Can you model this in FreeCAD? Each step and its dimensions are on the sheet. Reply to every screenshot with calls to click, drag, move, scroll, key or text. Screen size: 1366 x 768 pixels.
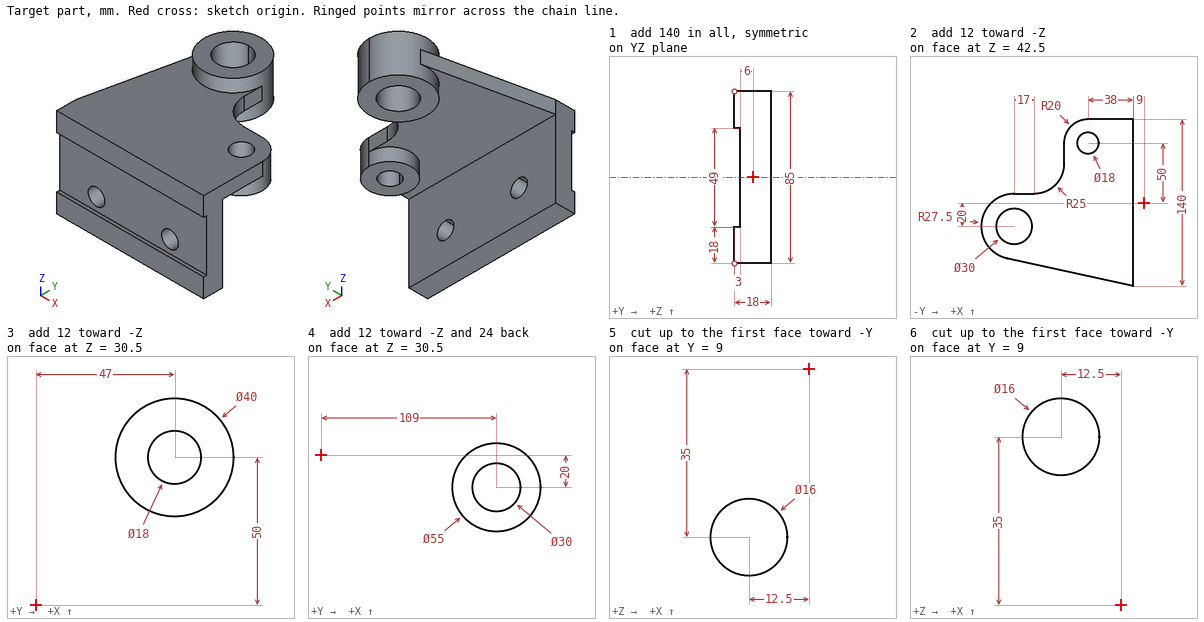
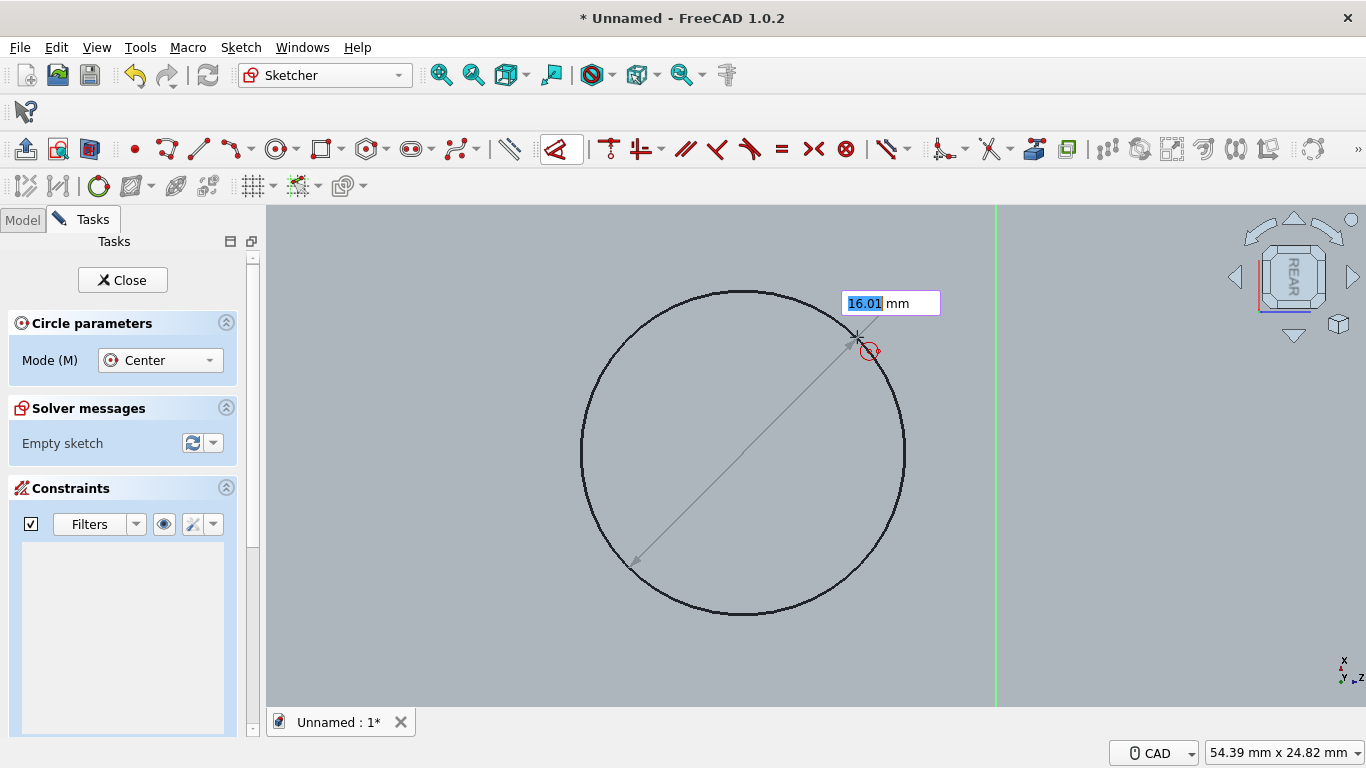
text(16)
key(Return)
key(Escape)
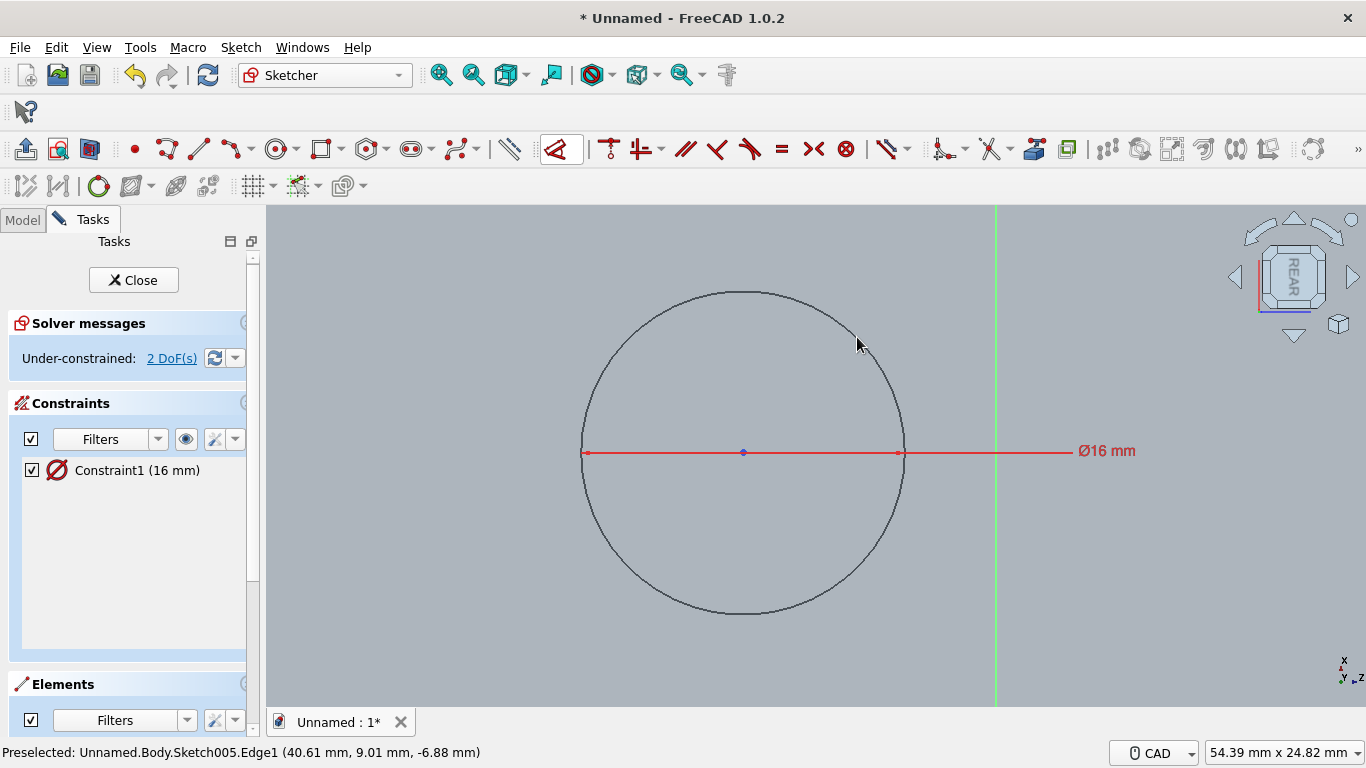
click(743, 453)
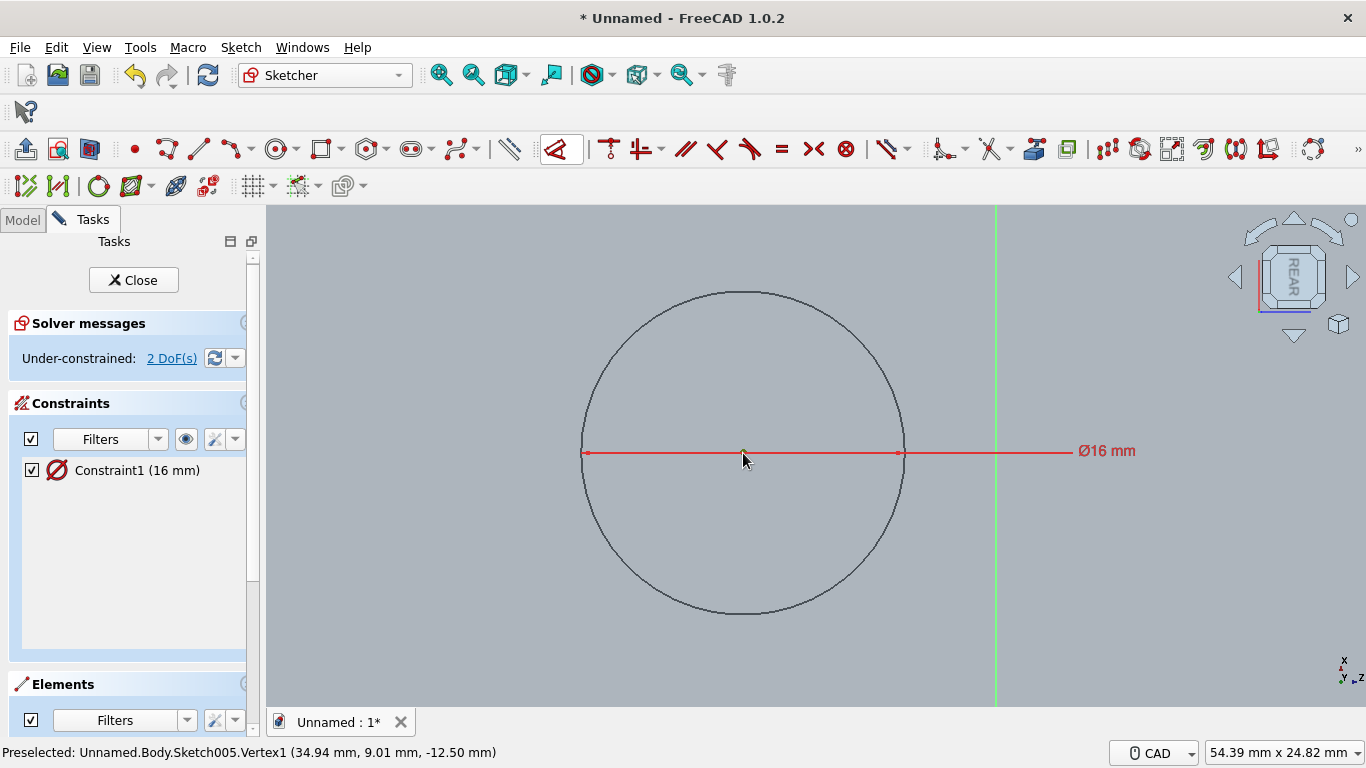
key(i)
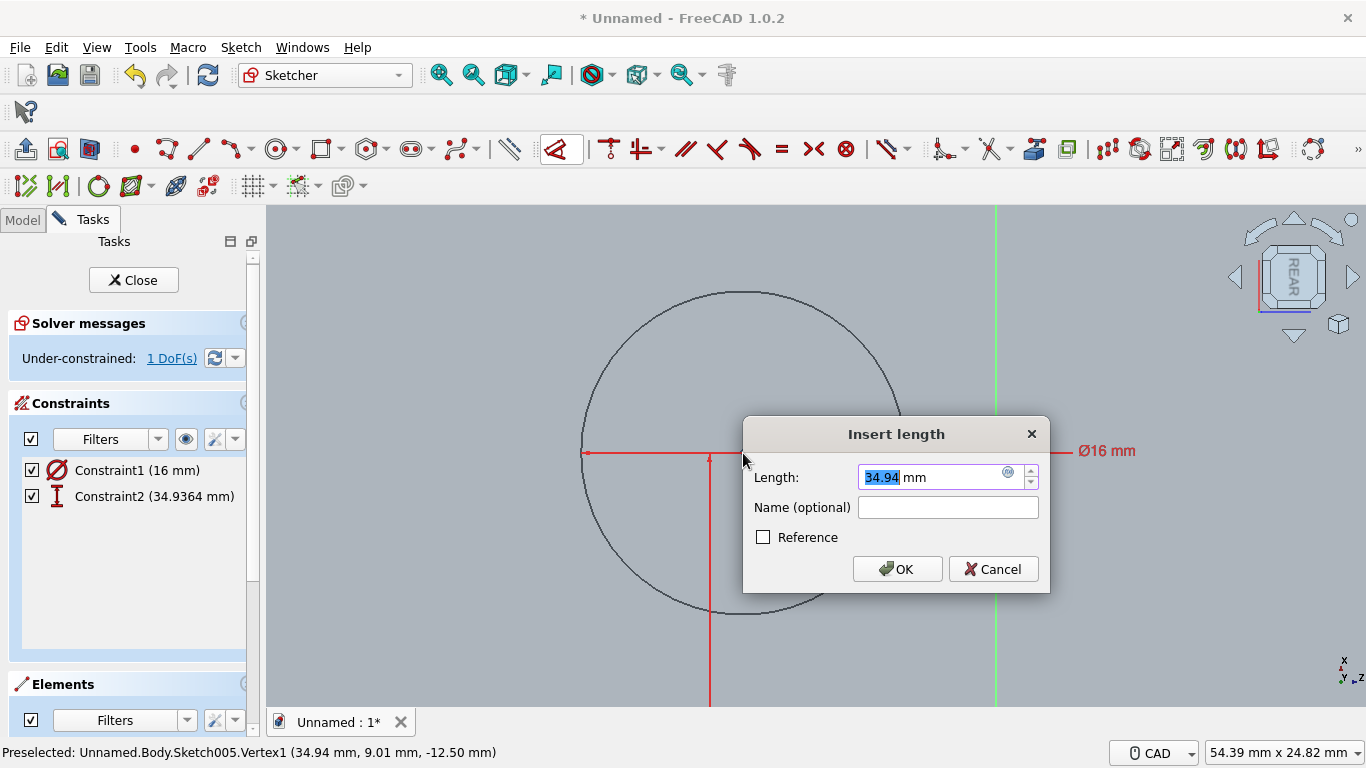
text(35)
key(Return)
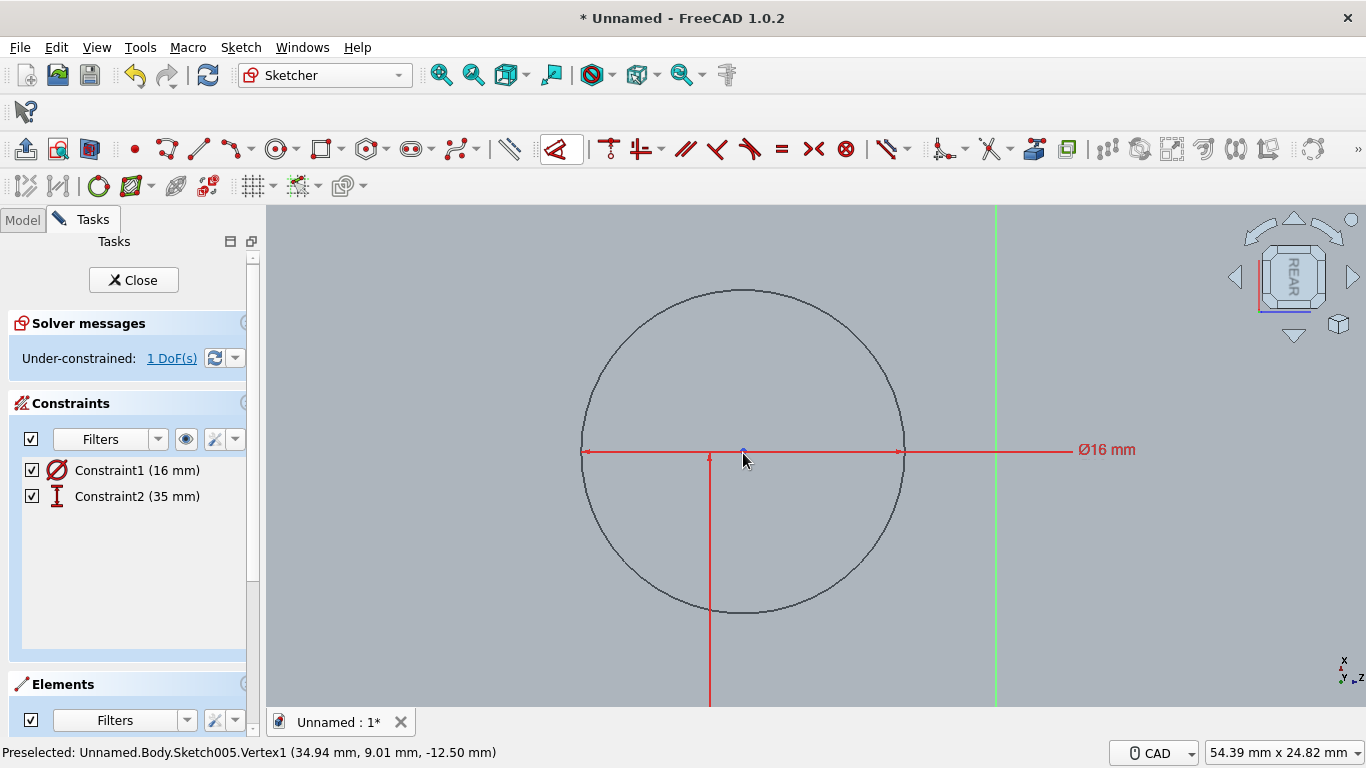
click(743, 452)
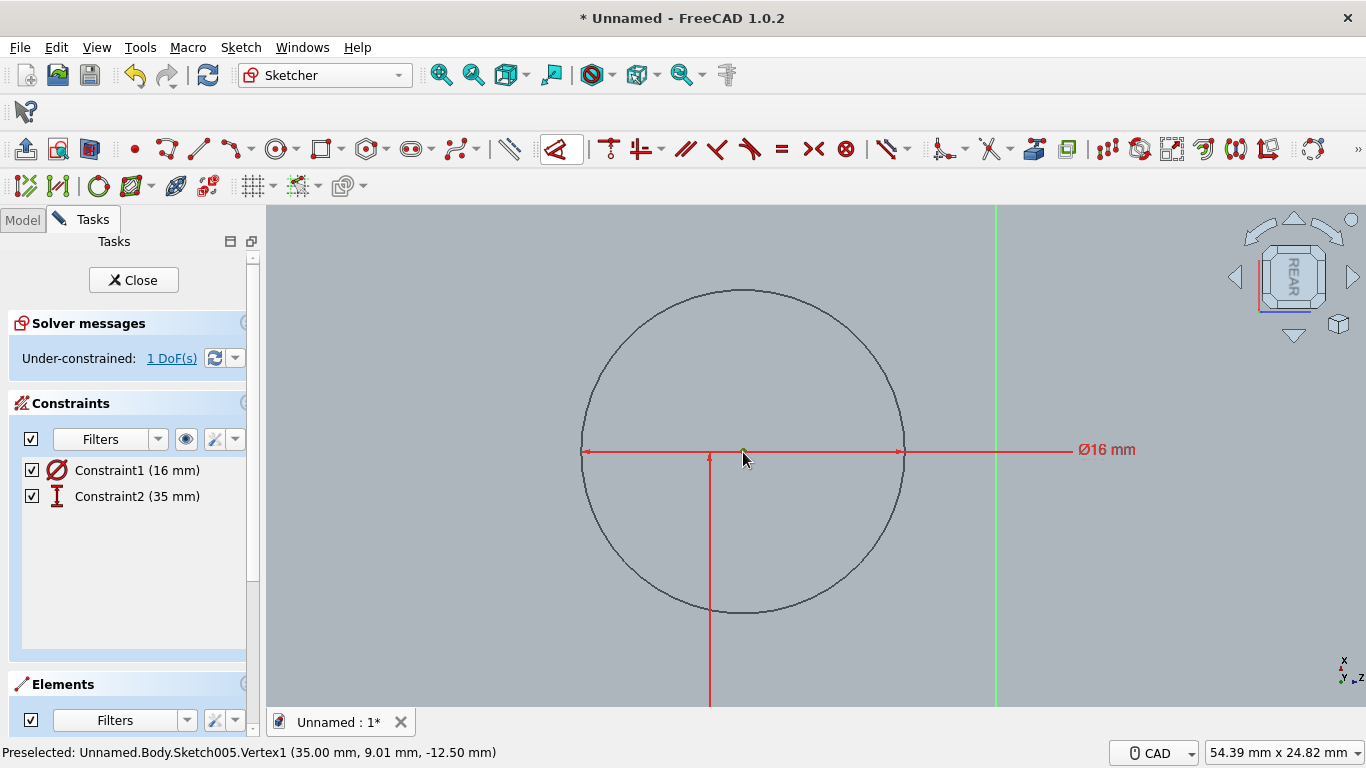
key(l)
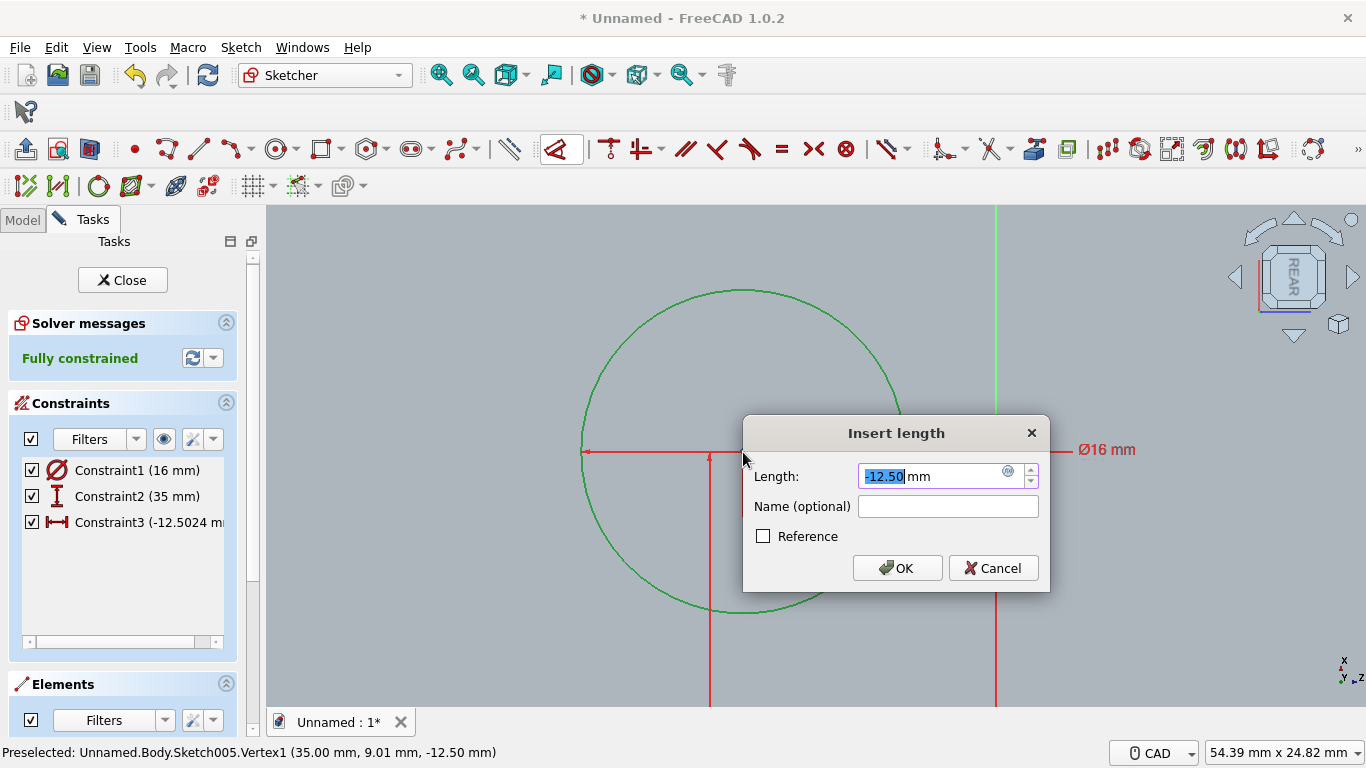
text(-12.5)
key(Return)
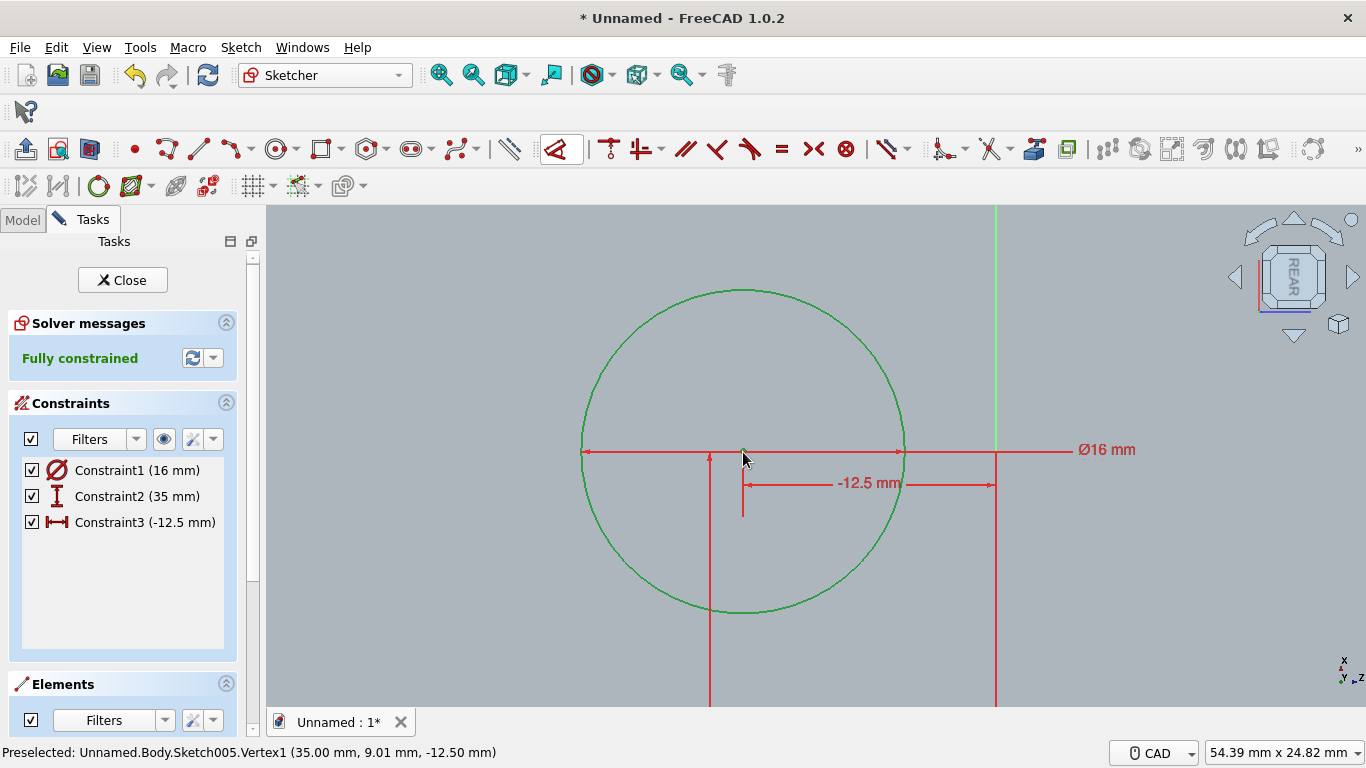
click(123, 280)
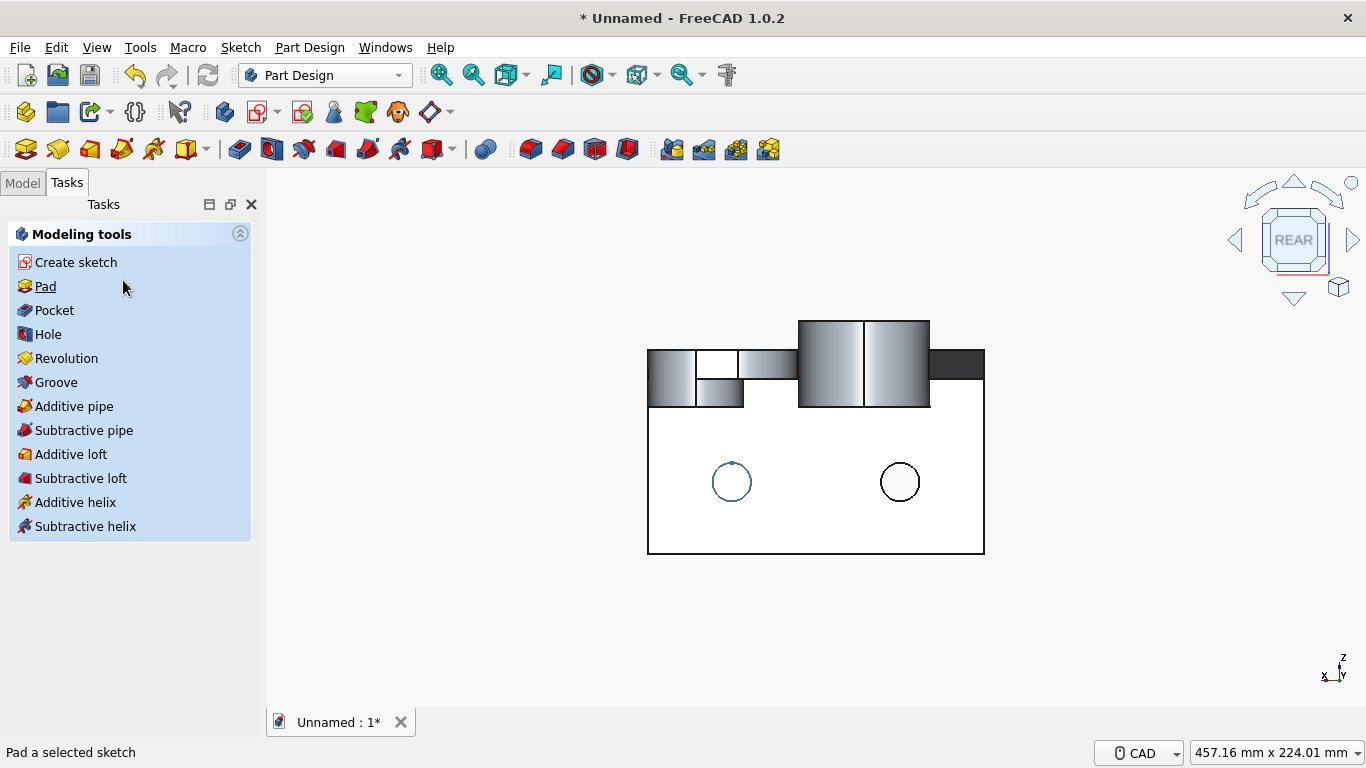
click(240, 150)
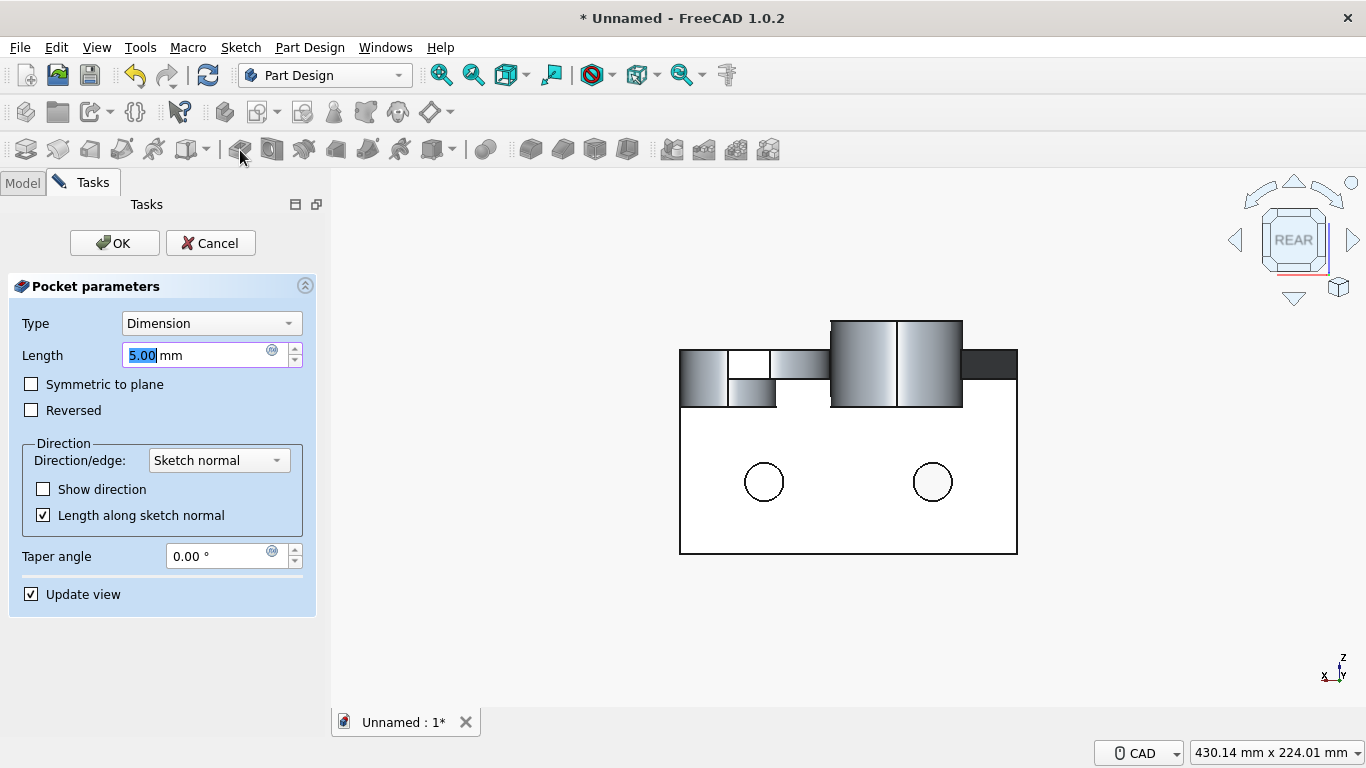
click(212, 324)